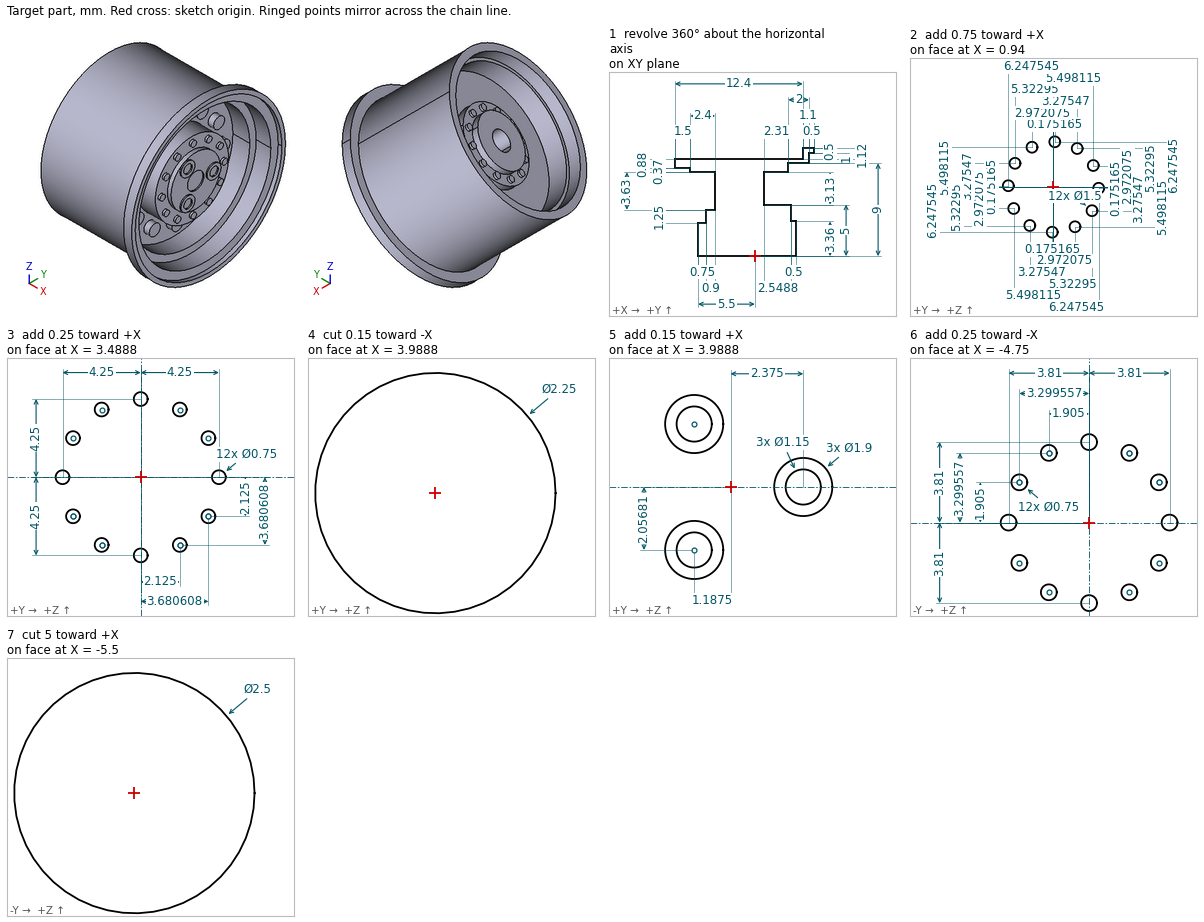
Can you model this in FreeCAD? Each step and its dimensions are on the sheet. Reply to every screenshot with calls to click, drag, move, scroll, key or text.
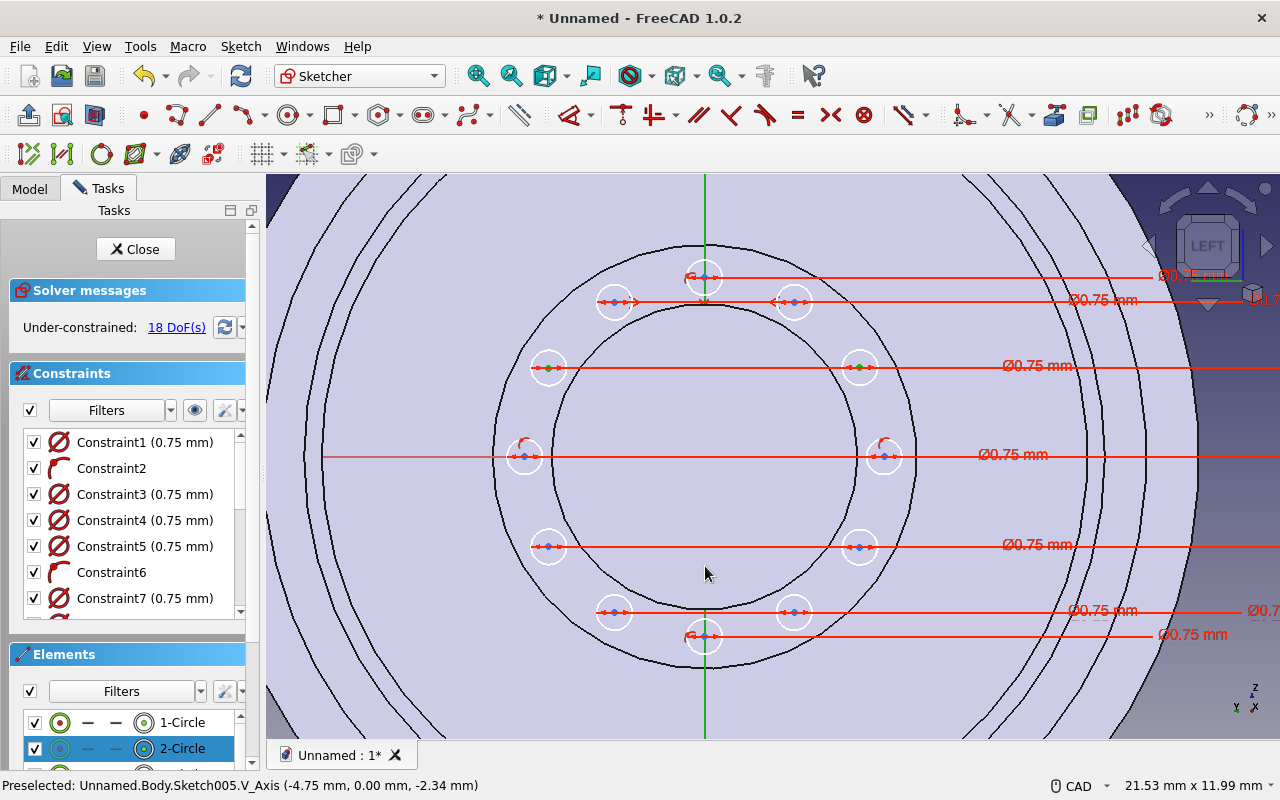
click(831, 116)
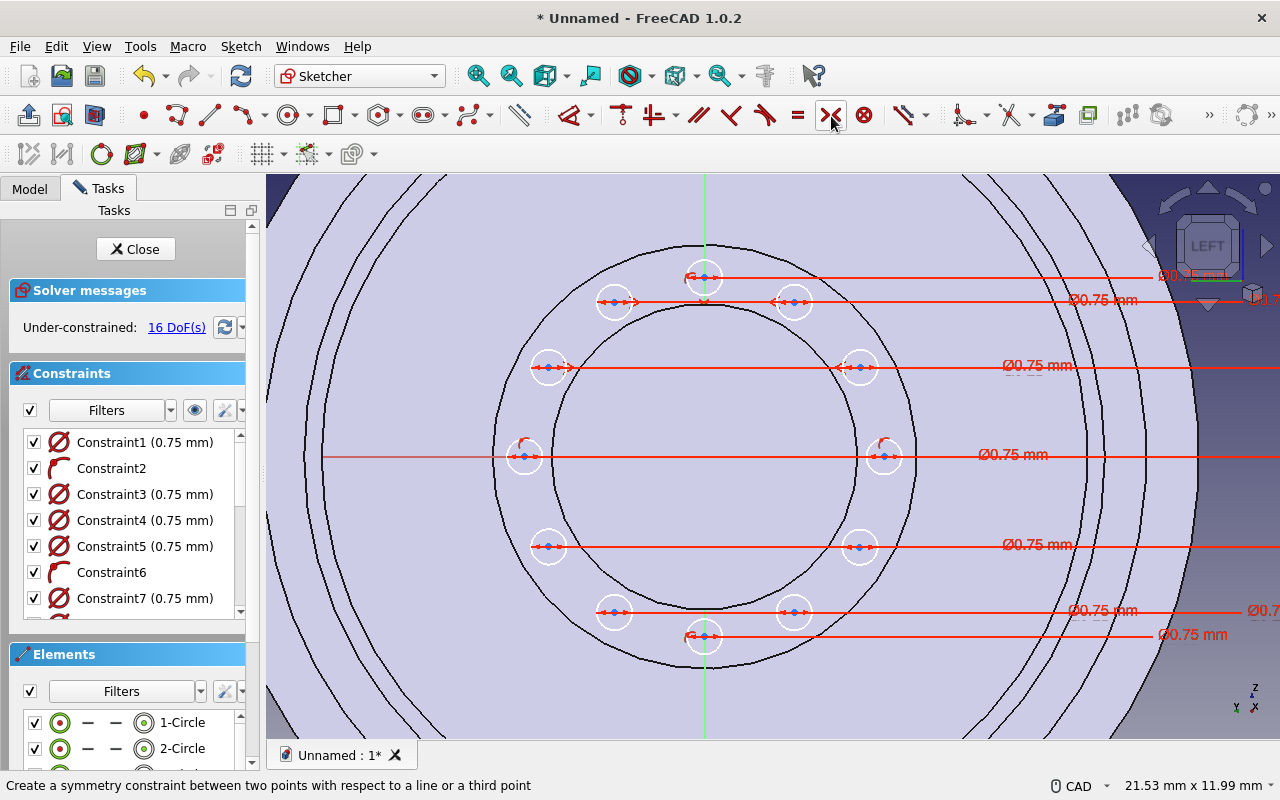
click(860, 368)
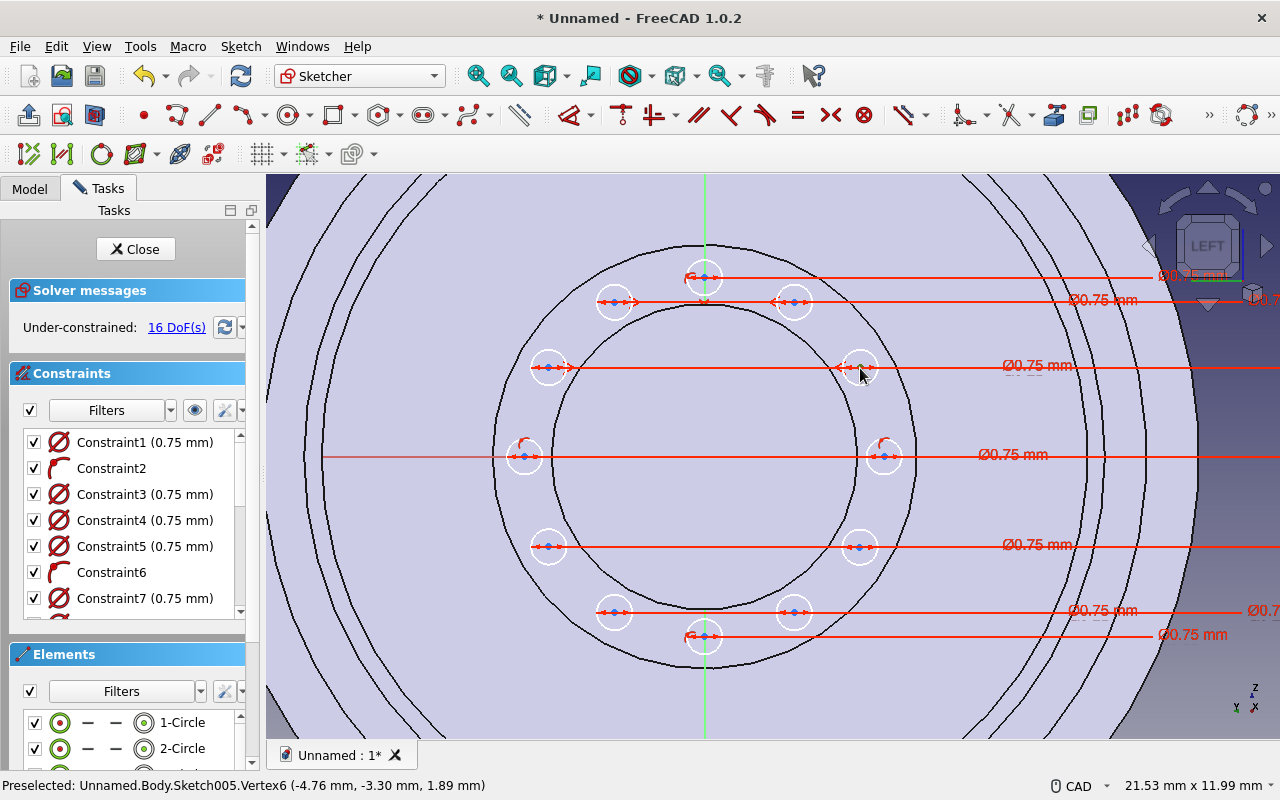
click(860, 547)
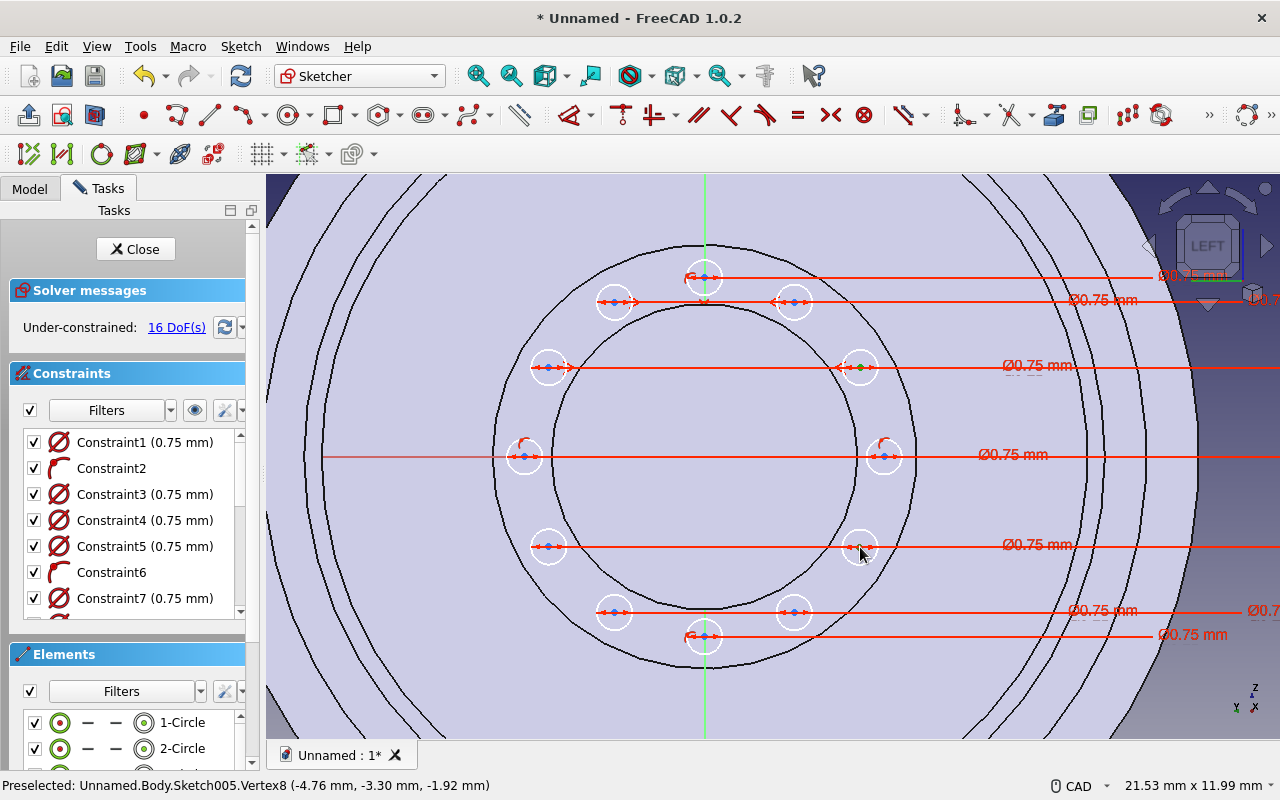
click(353, 457)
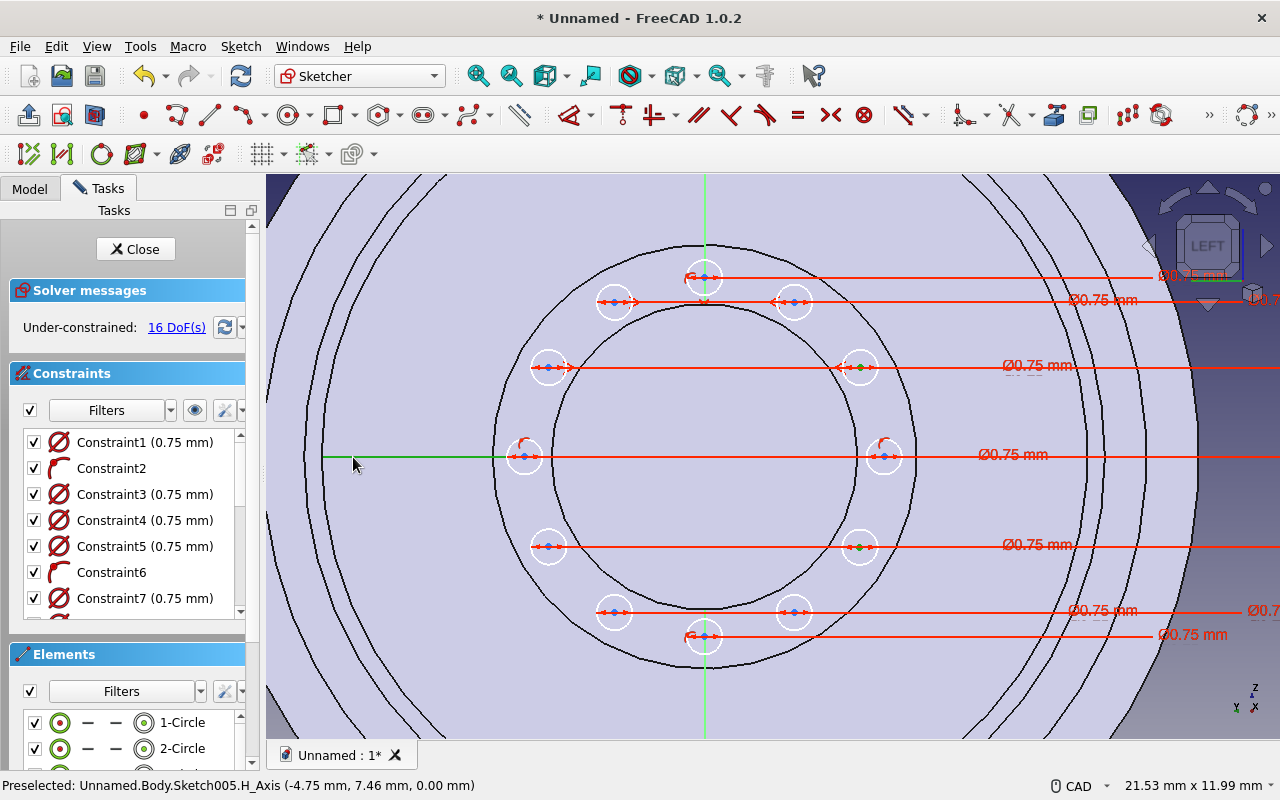
click(831, 116)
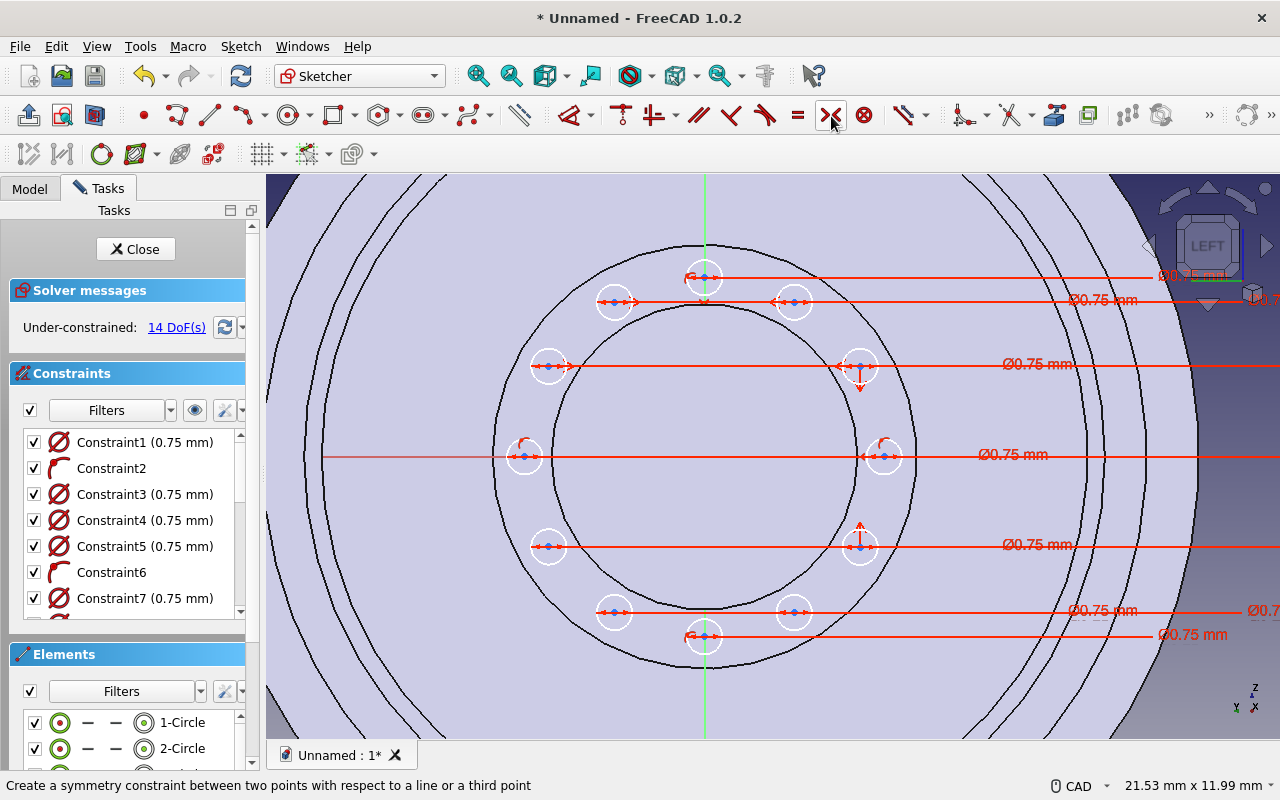
click(794, 302)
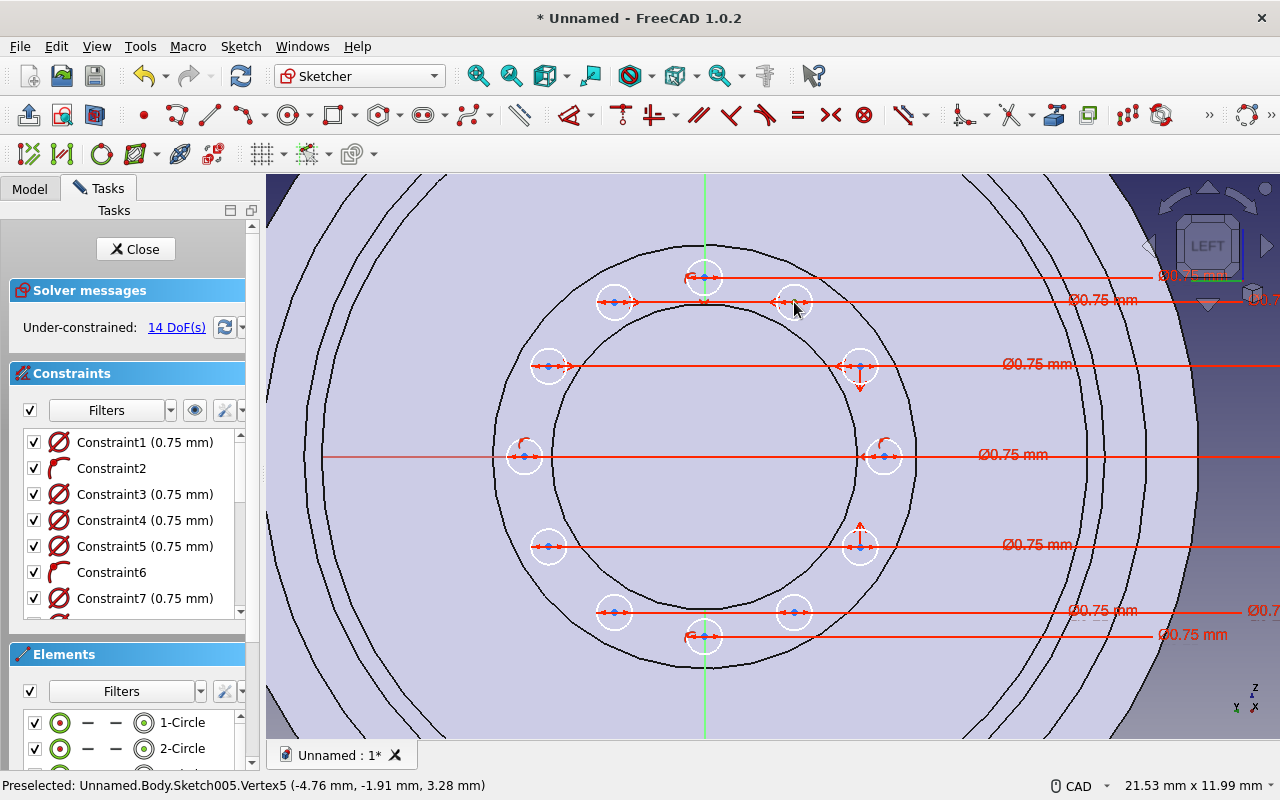
click(794, 613)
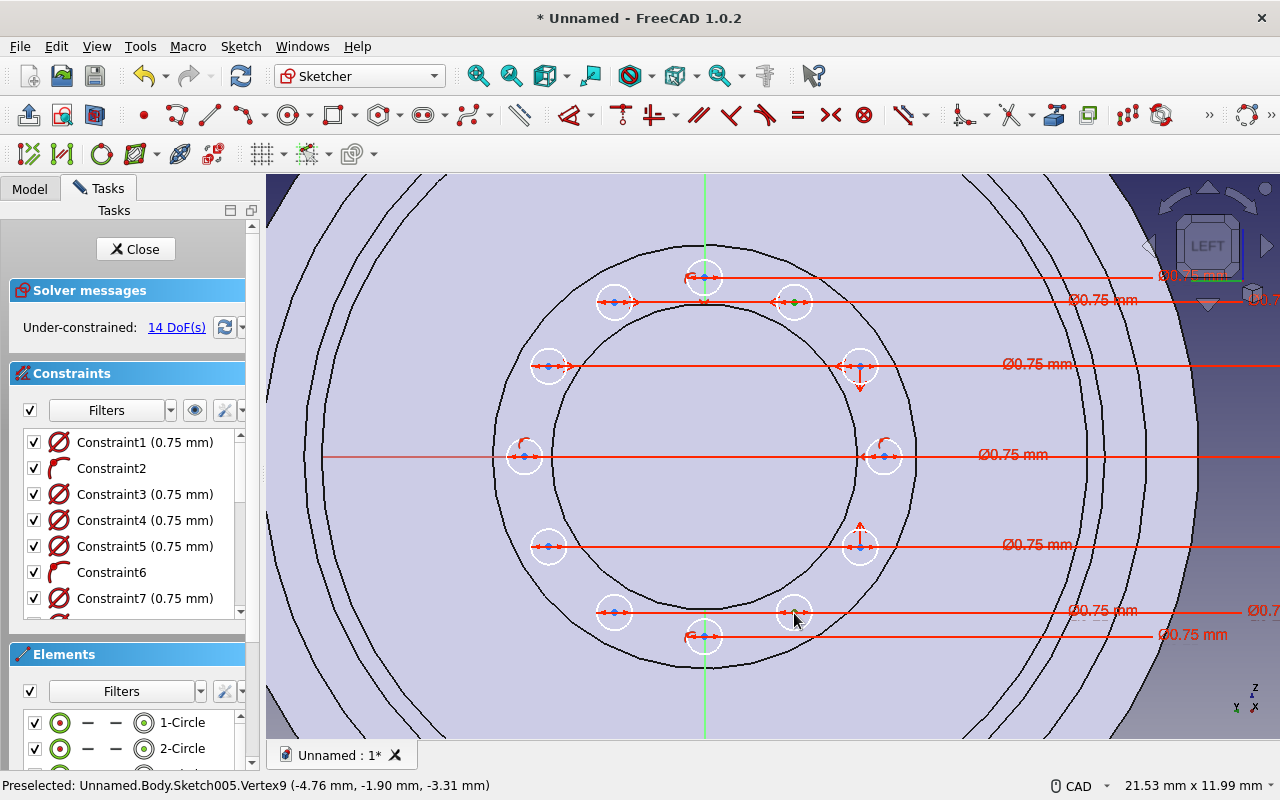
click(353, 457)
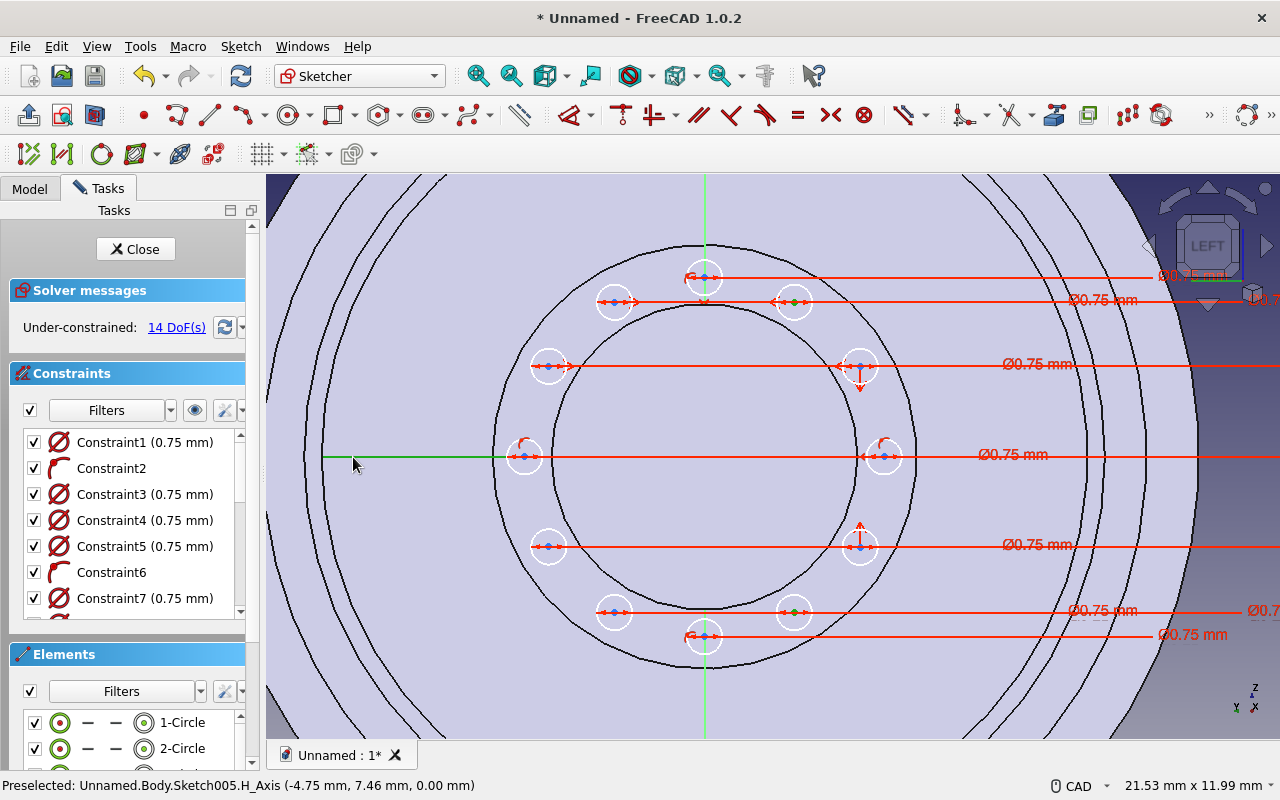
click(831, 116)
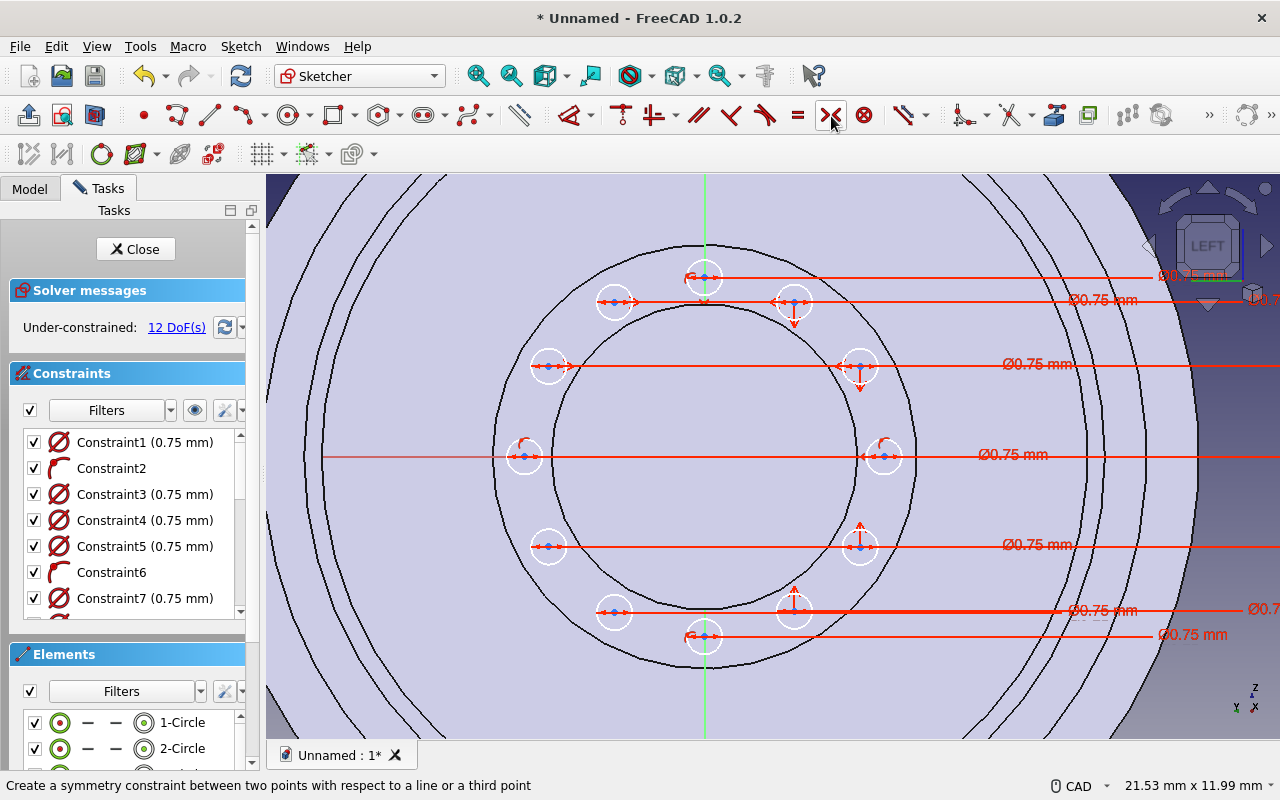
click(615, 302)